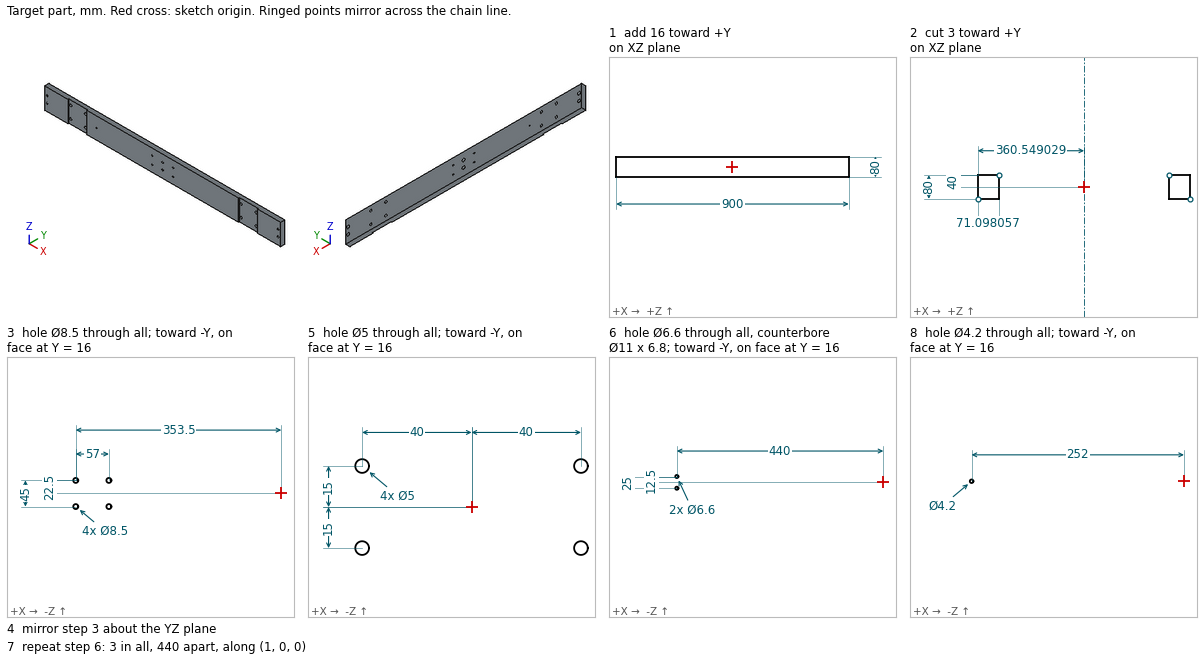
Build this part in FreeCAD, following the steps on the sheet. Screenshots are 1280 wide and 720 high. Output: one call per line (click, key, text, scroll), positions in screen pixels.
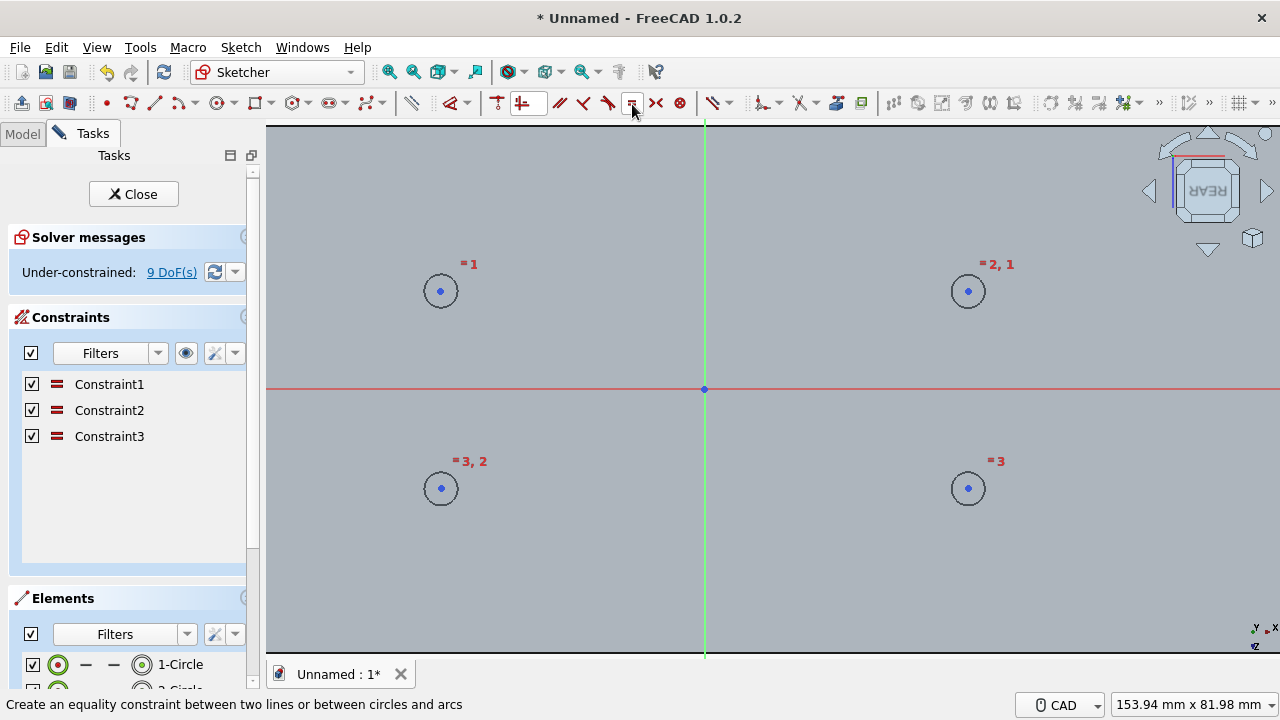
click(441, 291)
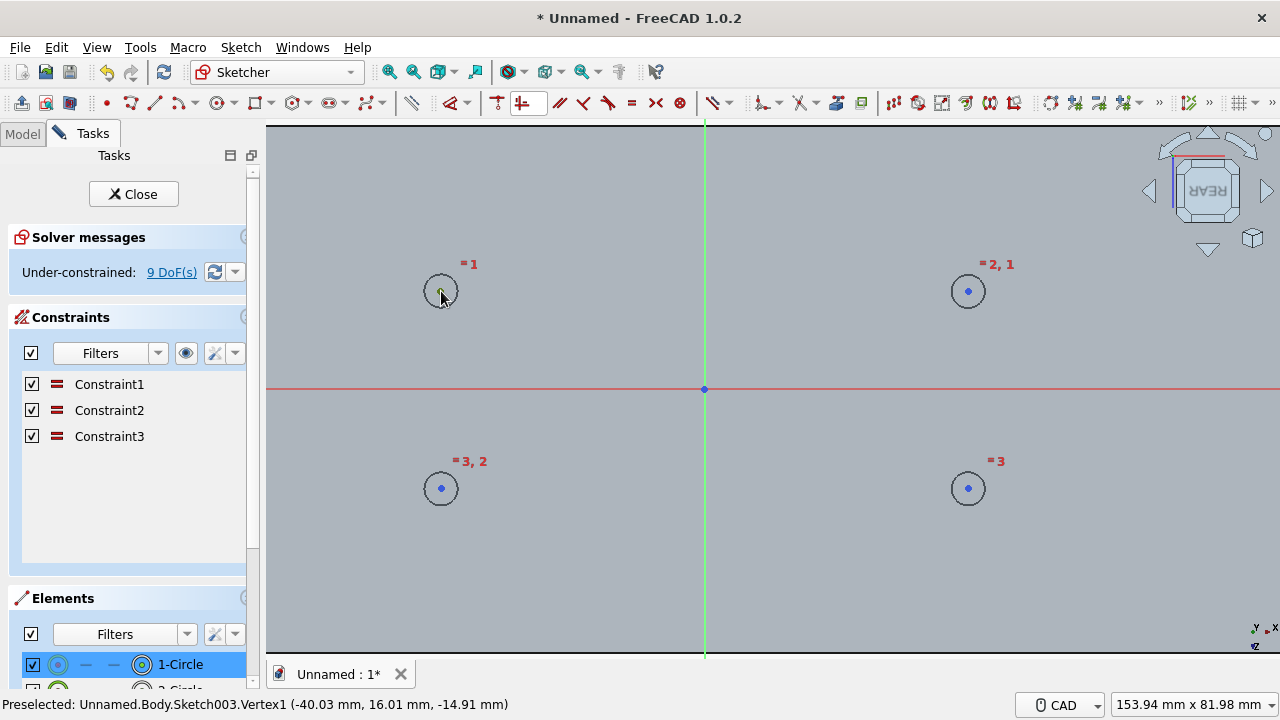
click(968, 291)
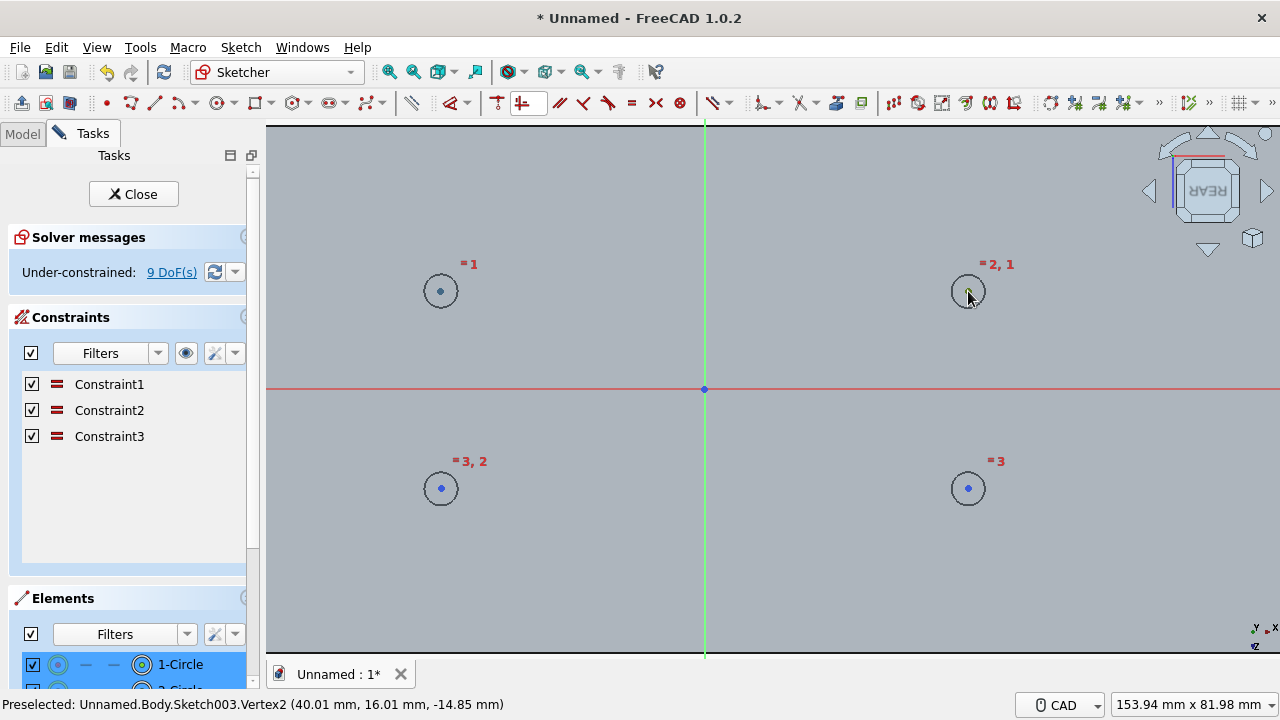
key(h)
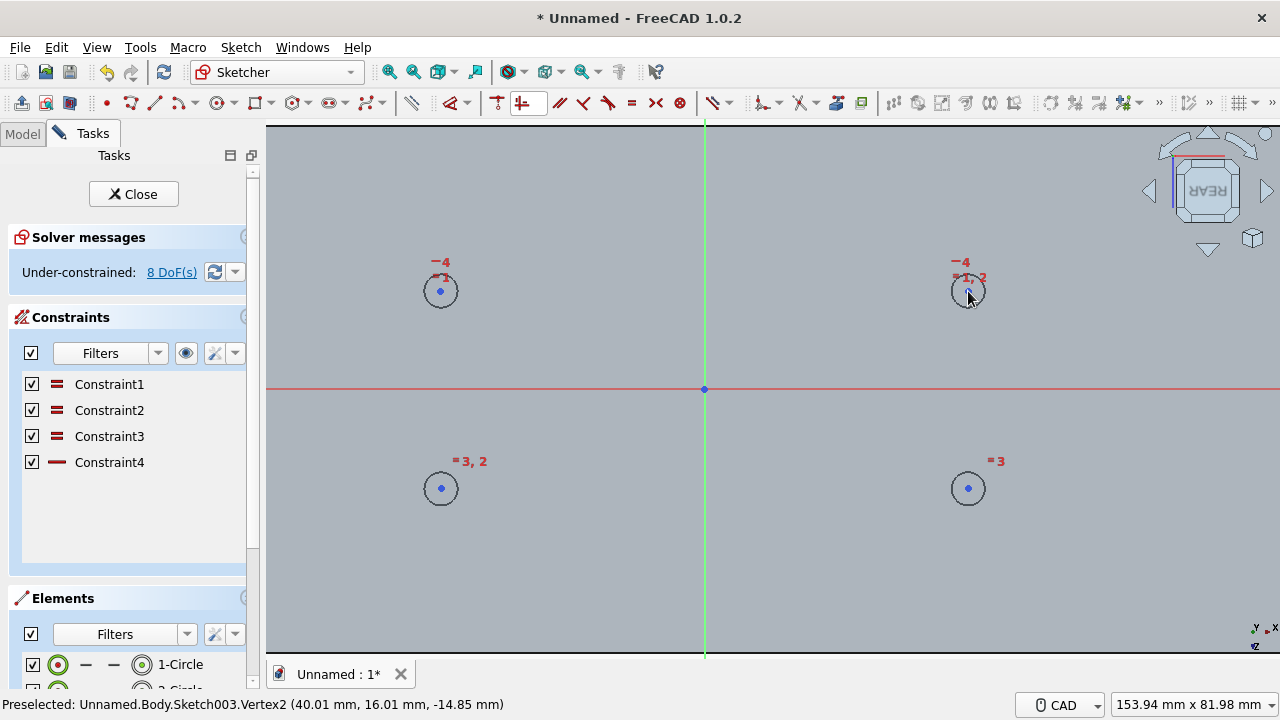
click(441, 291)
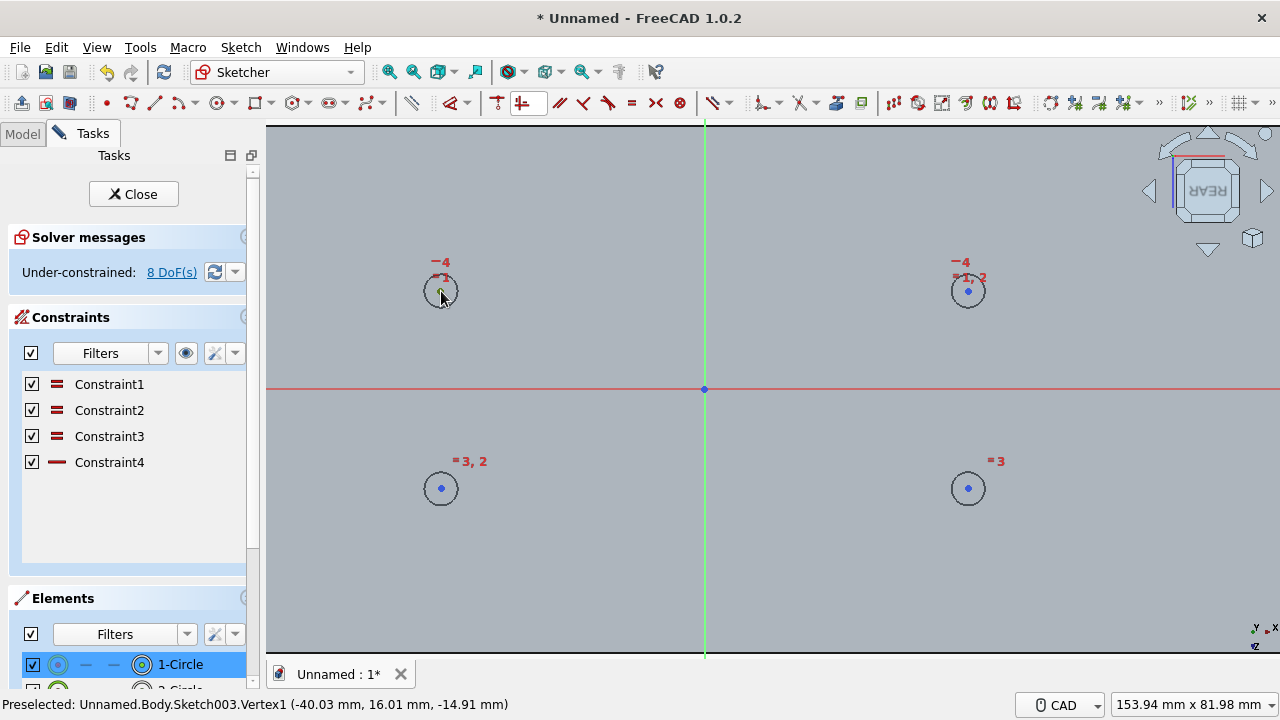
click(441, 489)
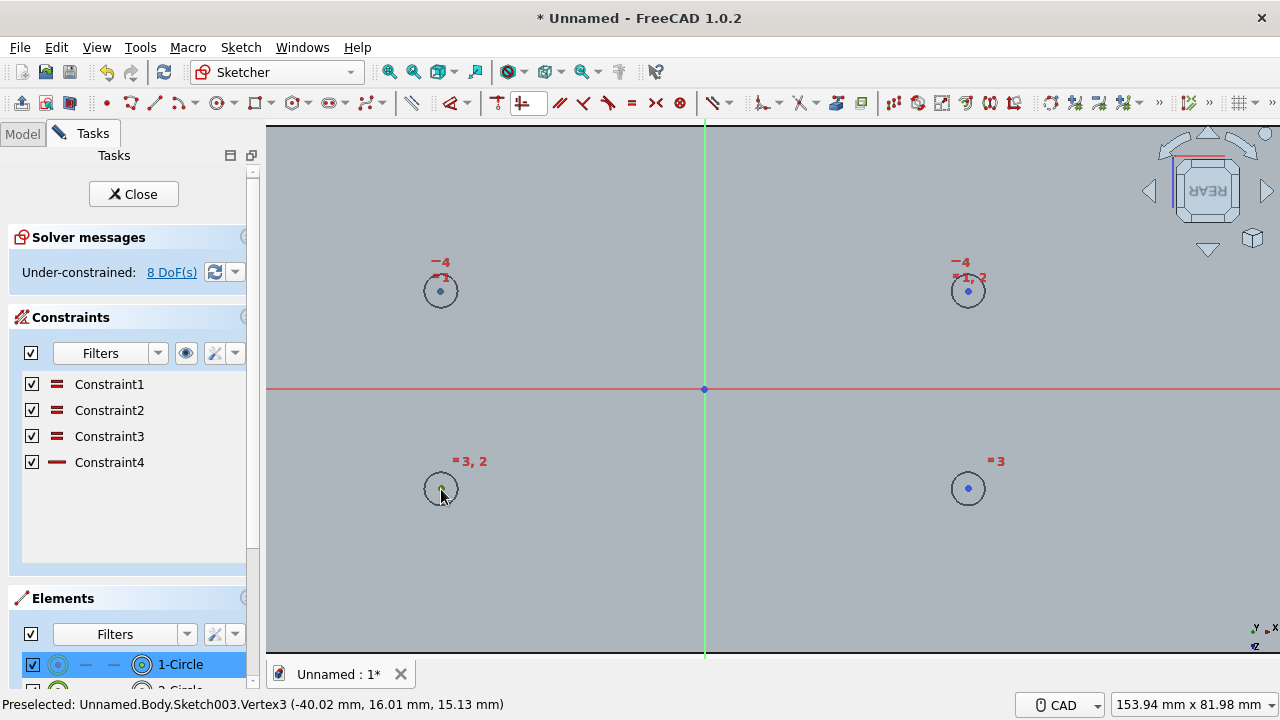
click(542, 104)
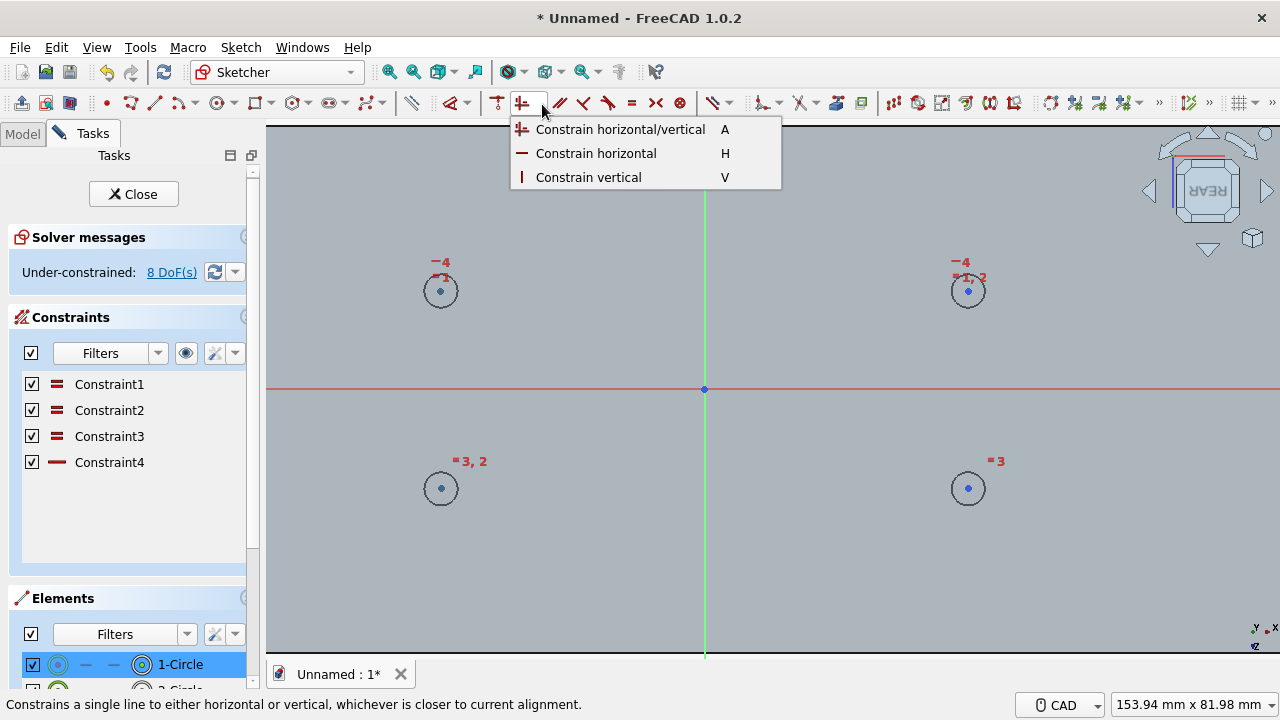
click(646, 177)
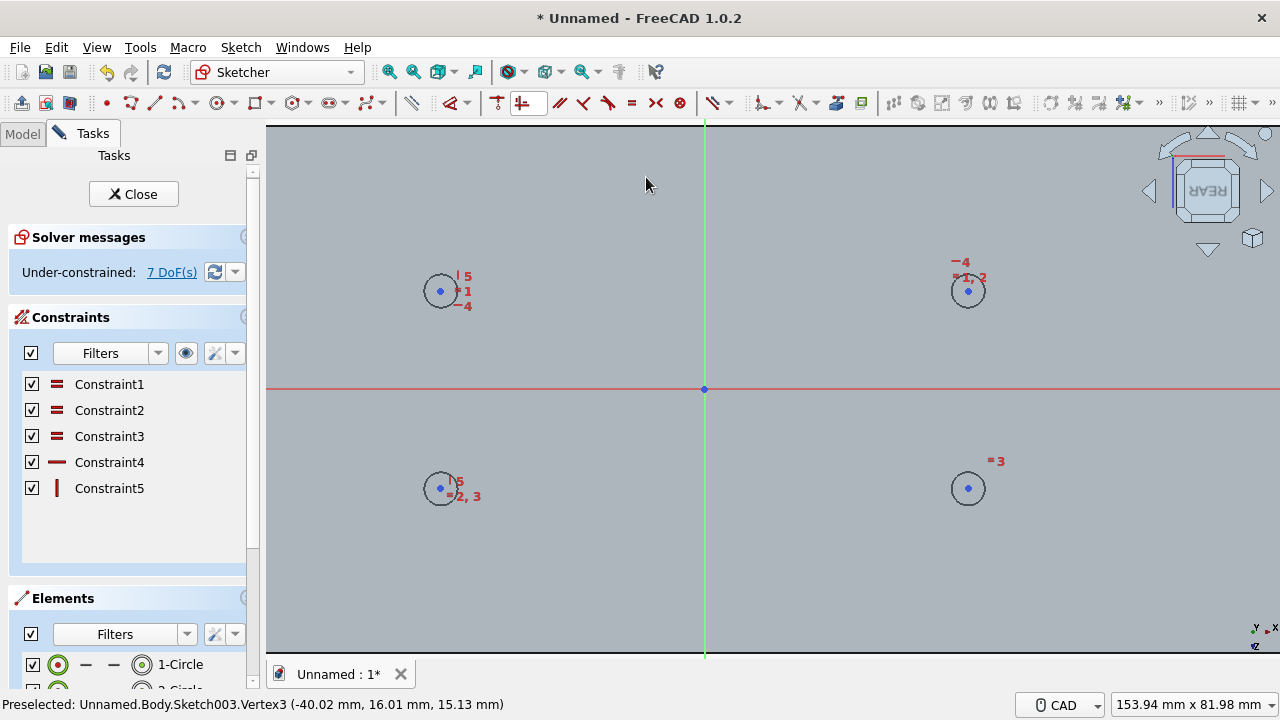
click(968, 291)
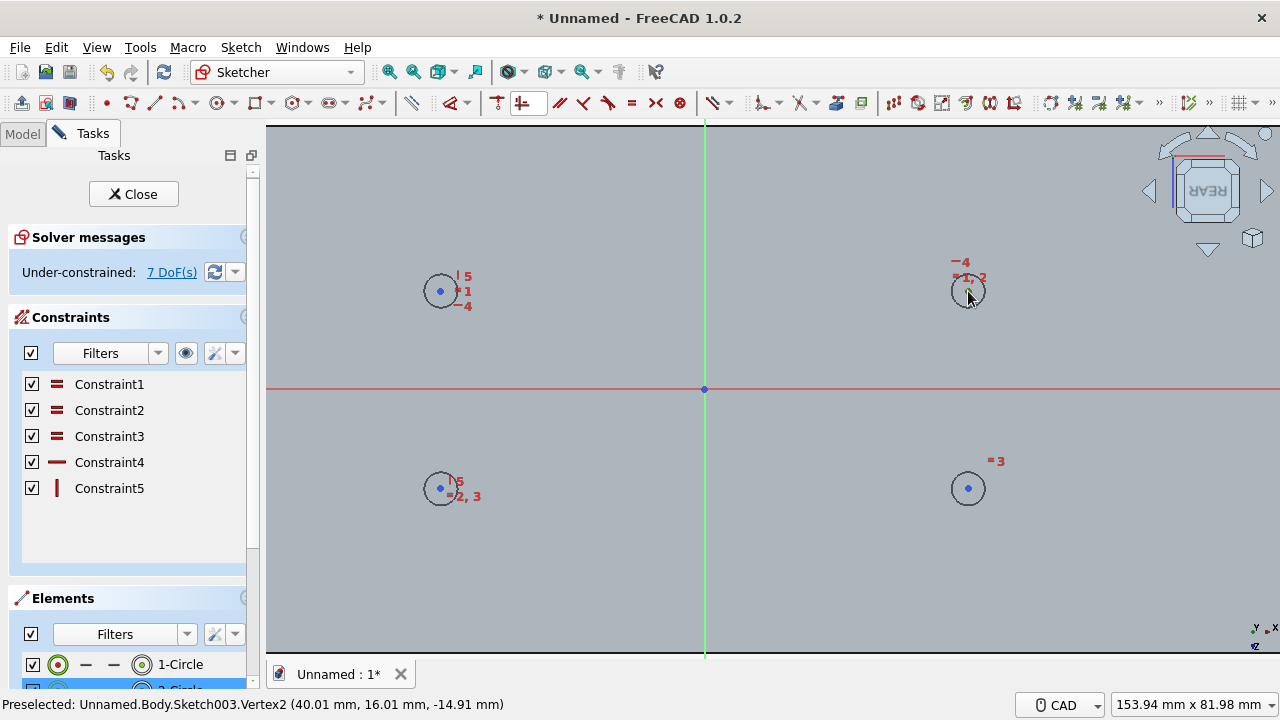
click(968, 489)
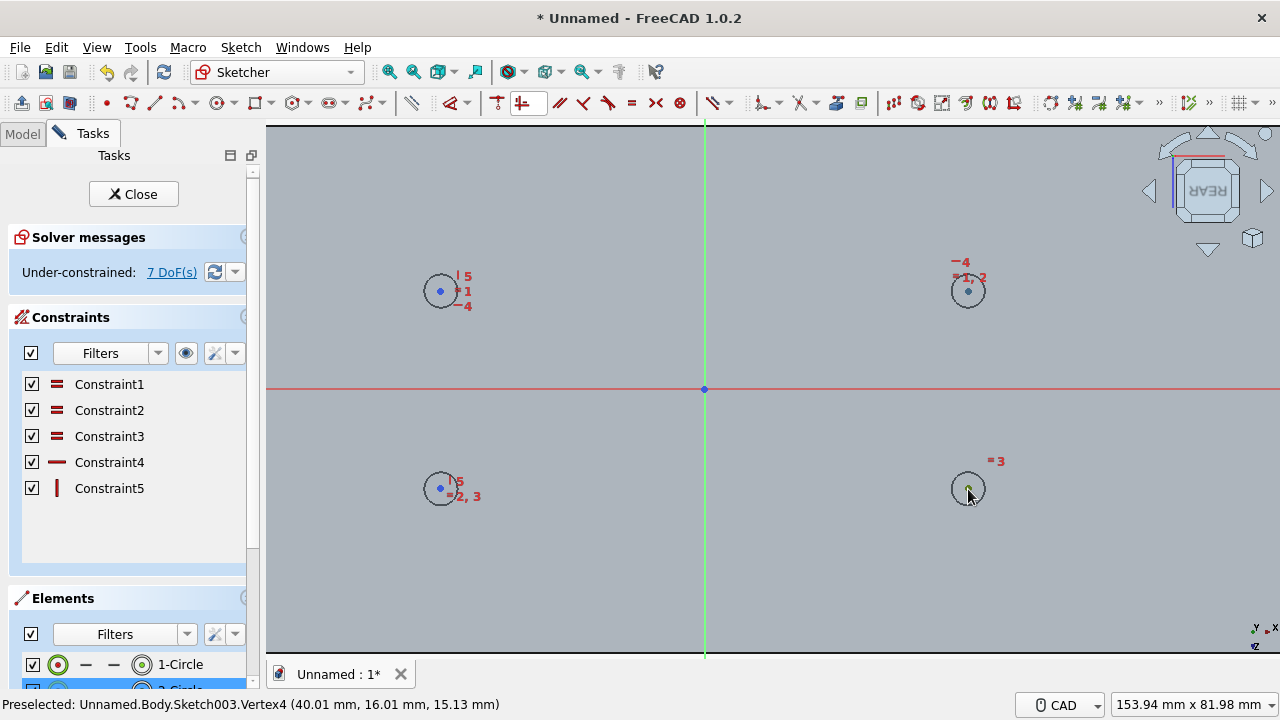
key(v)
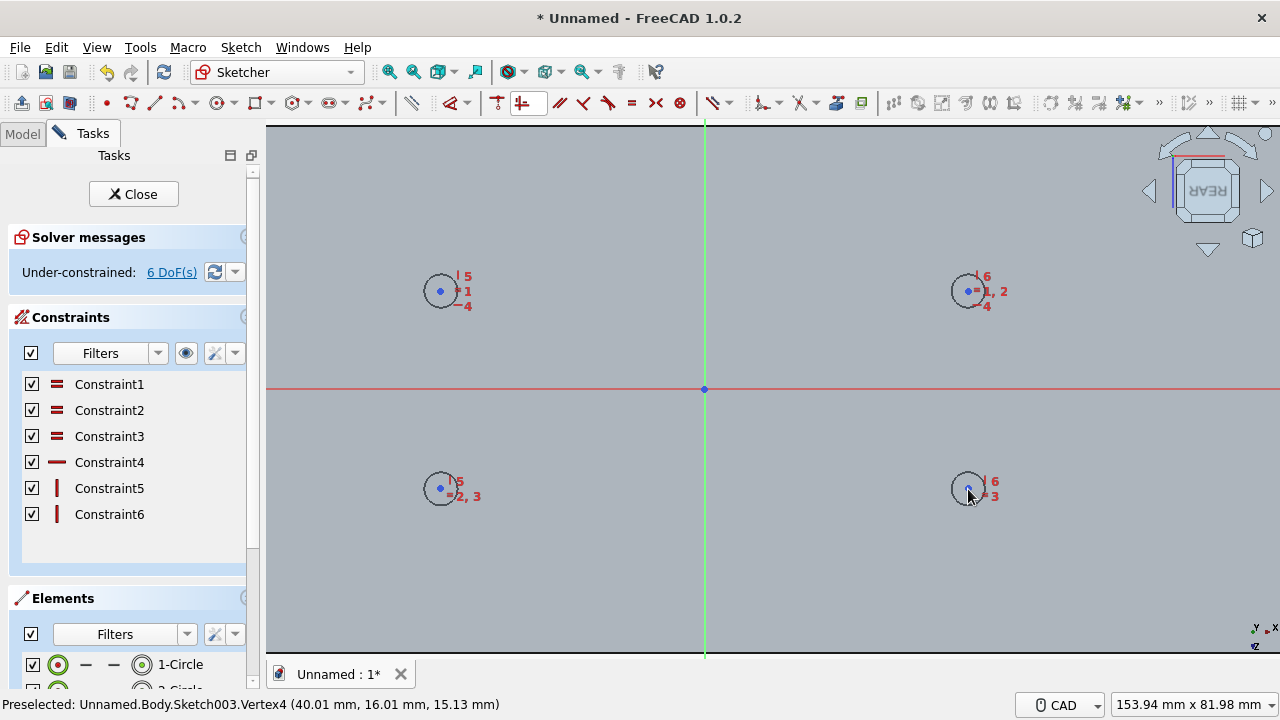
click(441, 489)